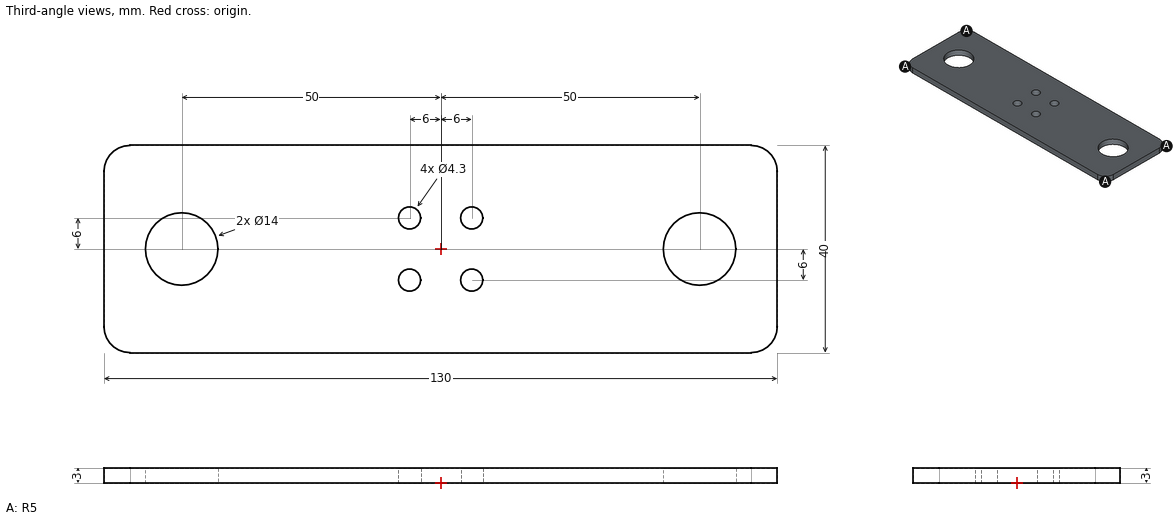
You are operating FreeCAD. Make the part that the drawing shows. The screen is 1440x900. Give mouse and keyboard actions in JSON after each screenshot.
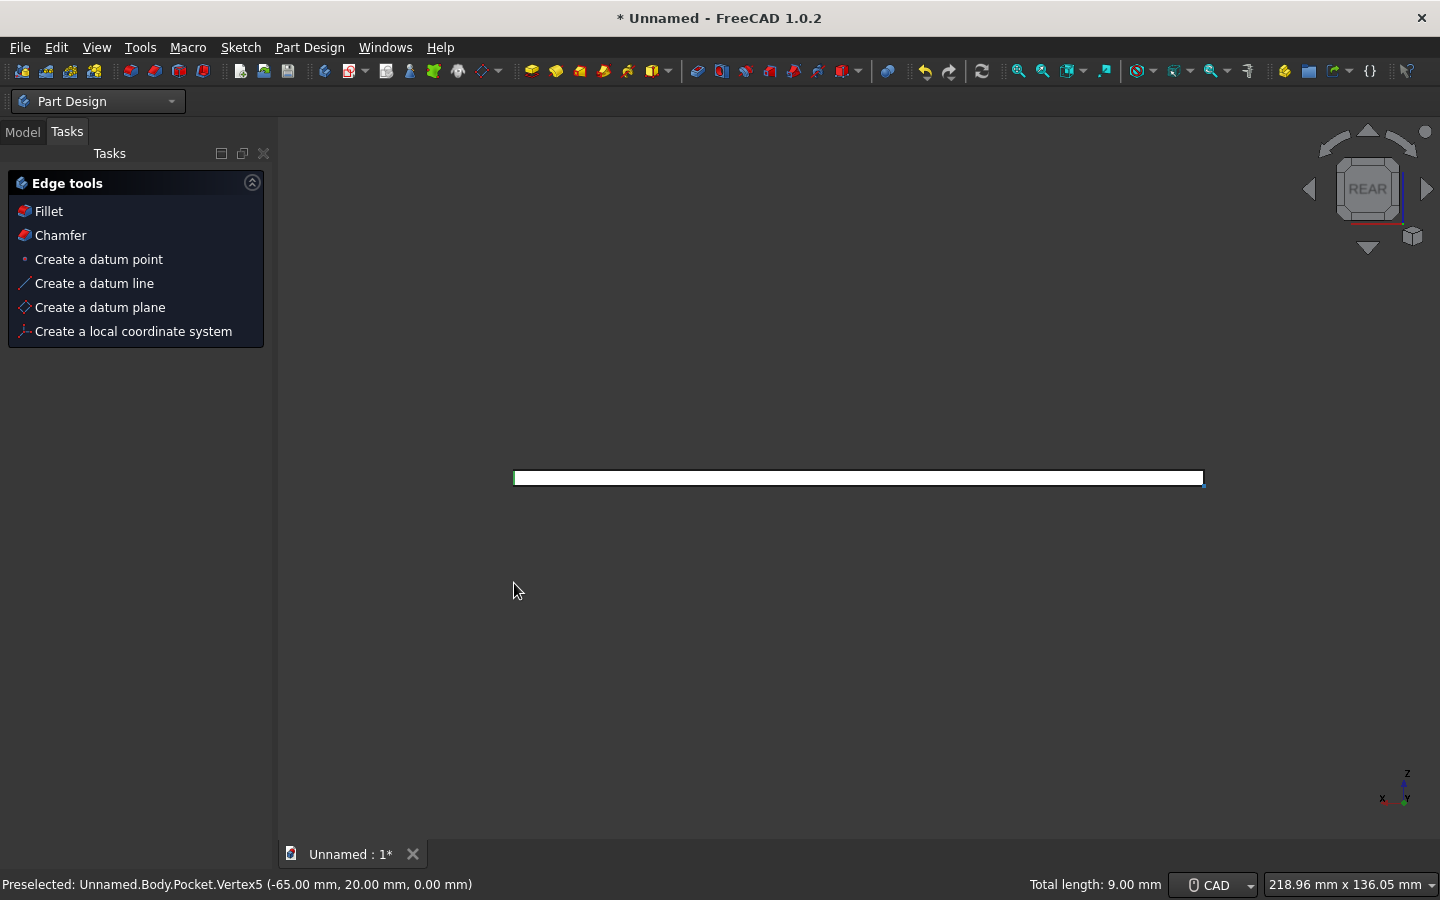
{"action": "left_click", "coordinate": [1204, 477], "text": "ctrl"}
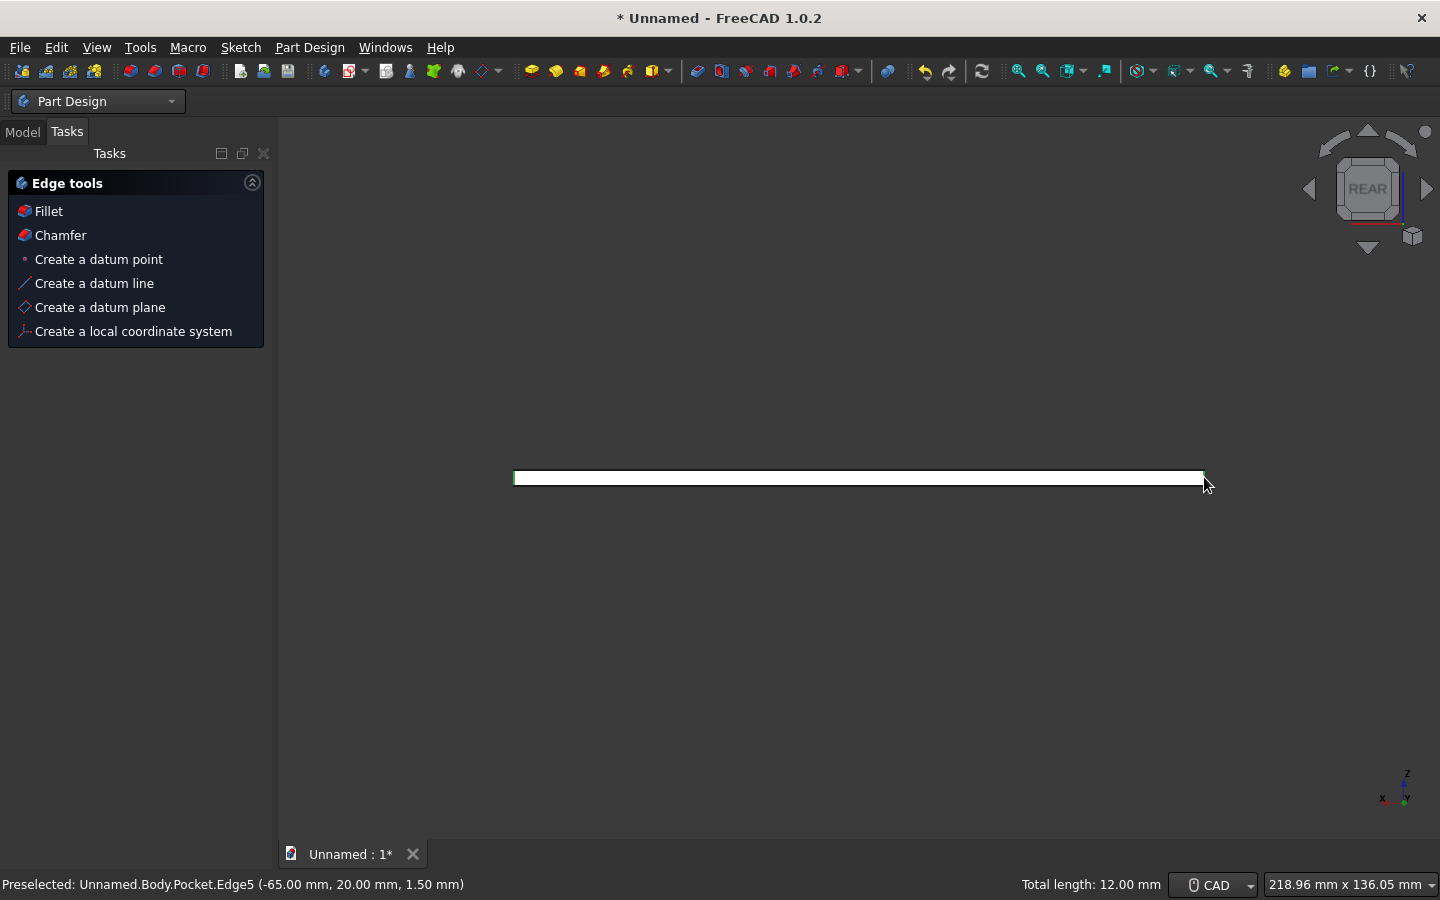
{"action": "left_click", "coordinate": [132, 72]}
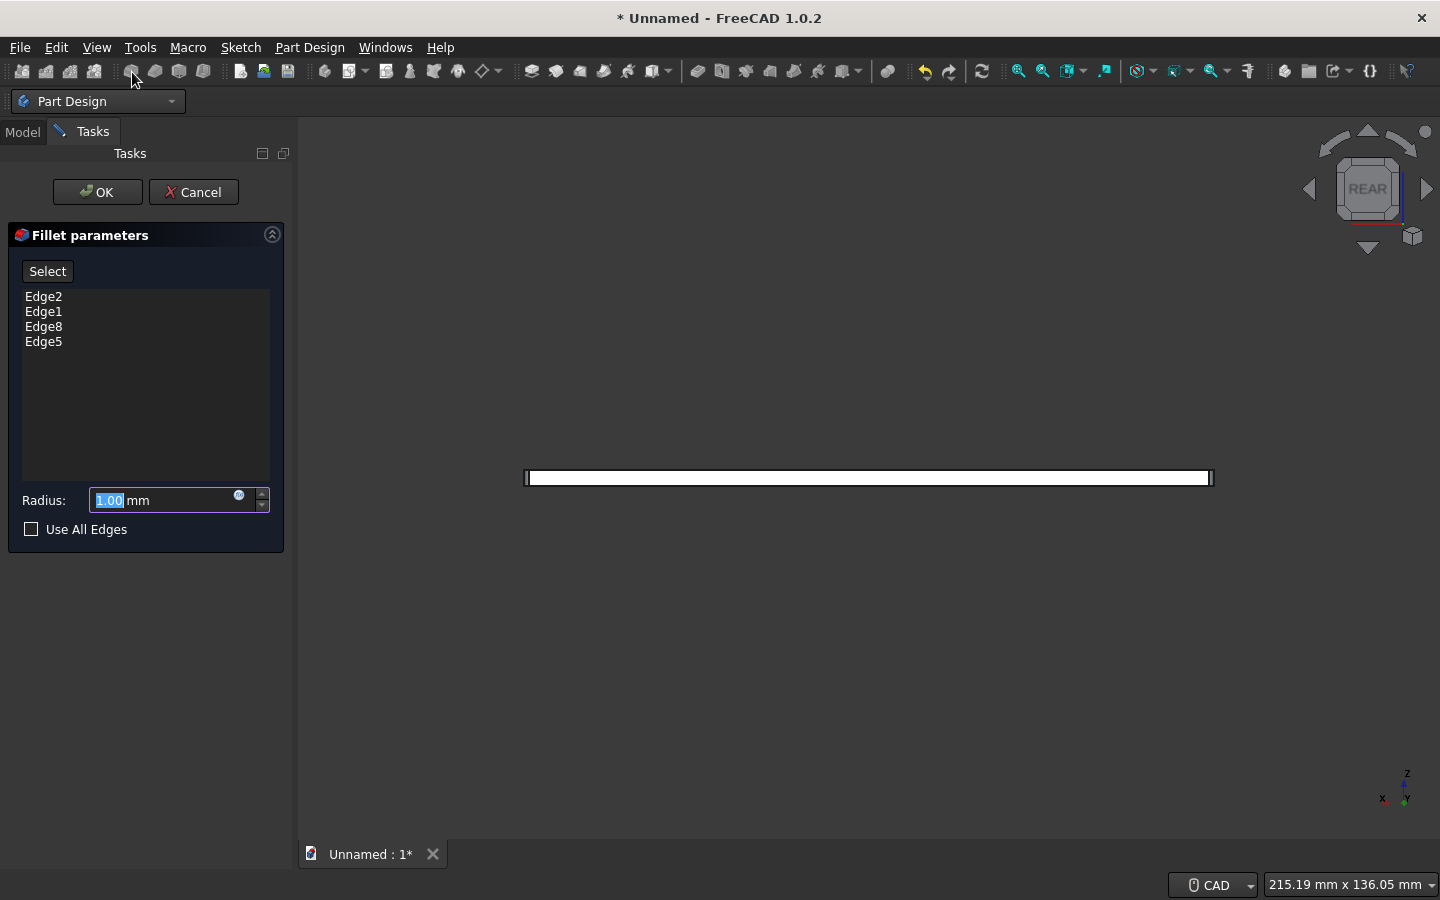
{"action": "type", "text": "5"}
{"action": "key", "text": "Tab"}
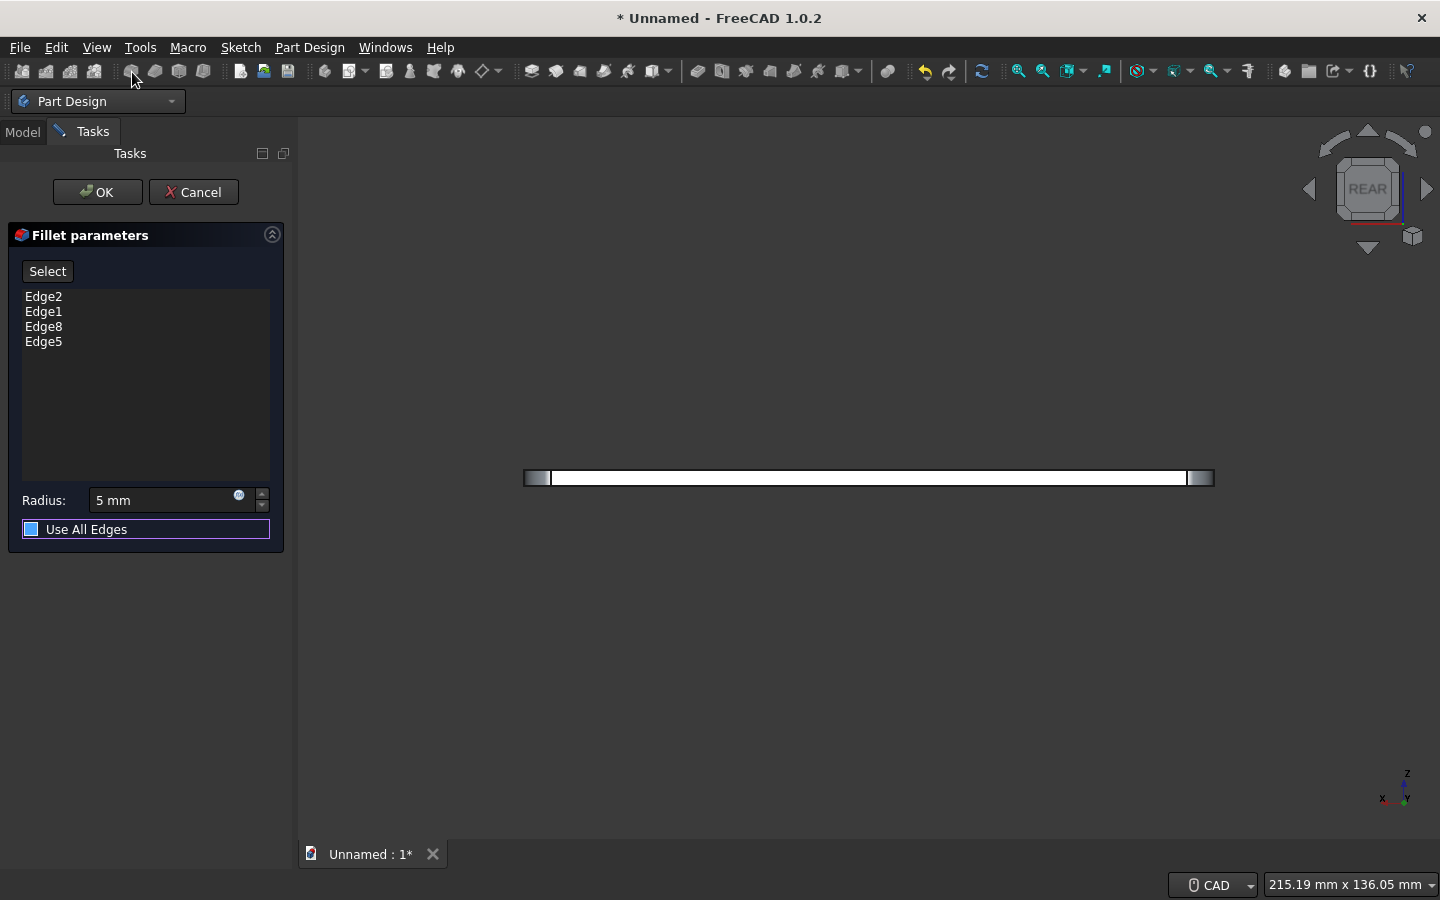
{"action": "left_click", "coordinate": [98, 192]}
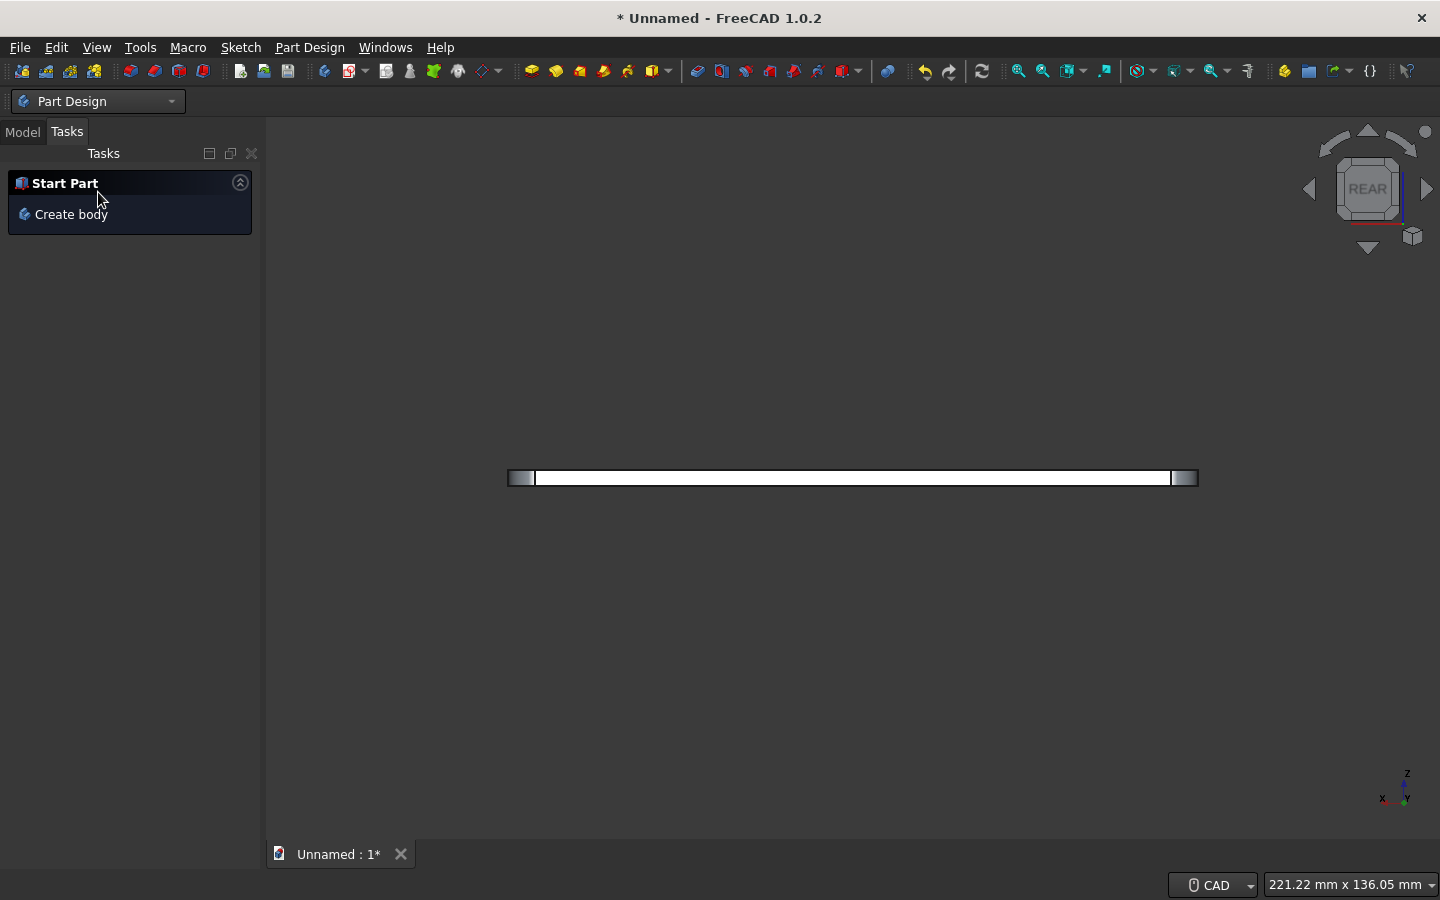
{"action": "key", "text": "0"}